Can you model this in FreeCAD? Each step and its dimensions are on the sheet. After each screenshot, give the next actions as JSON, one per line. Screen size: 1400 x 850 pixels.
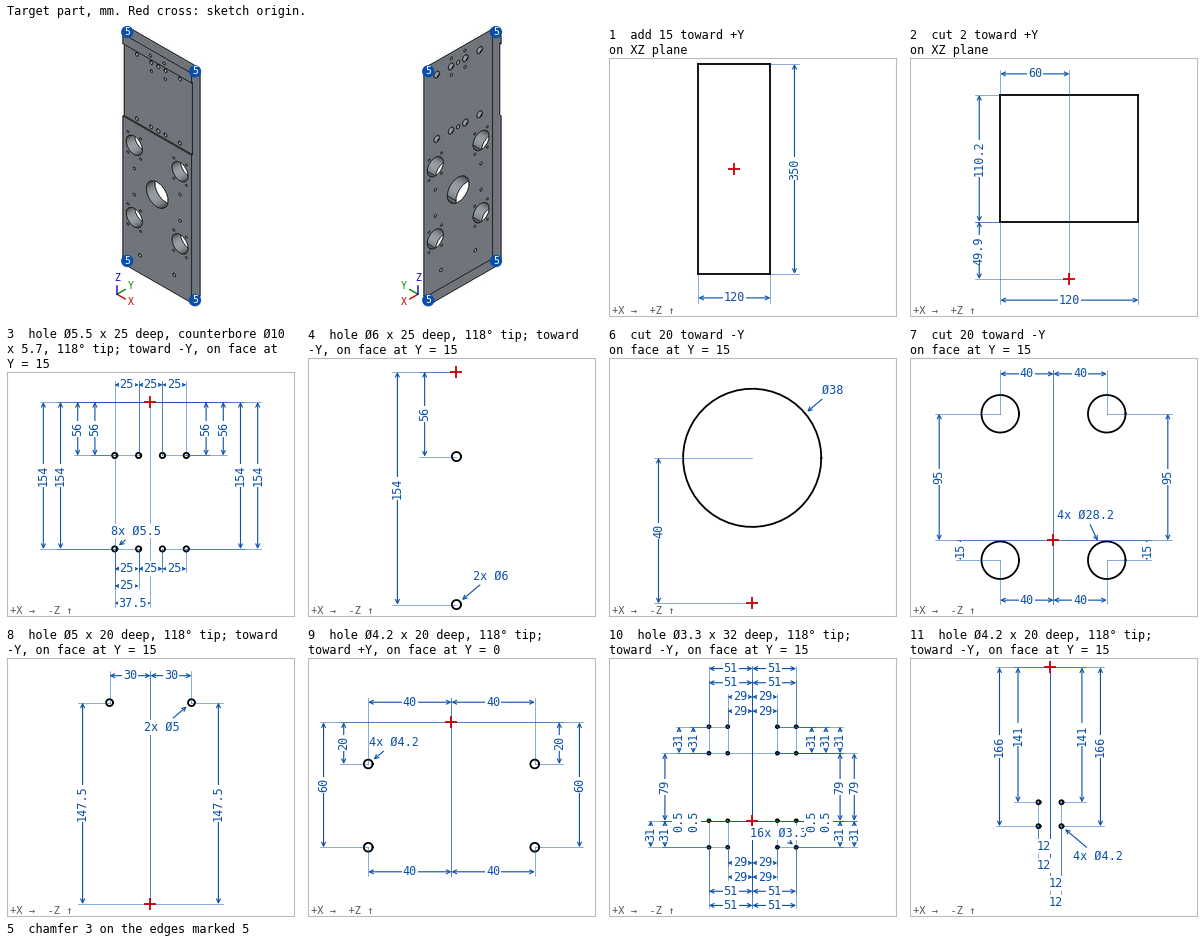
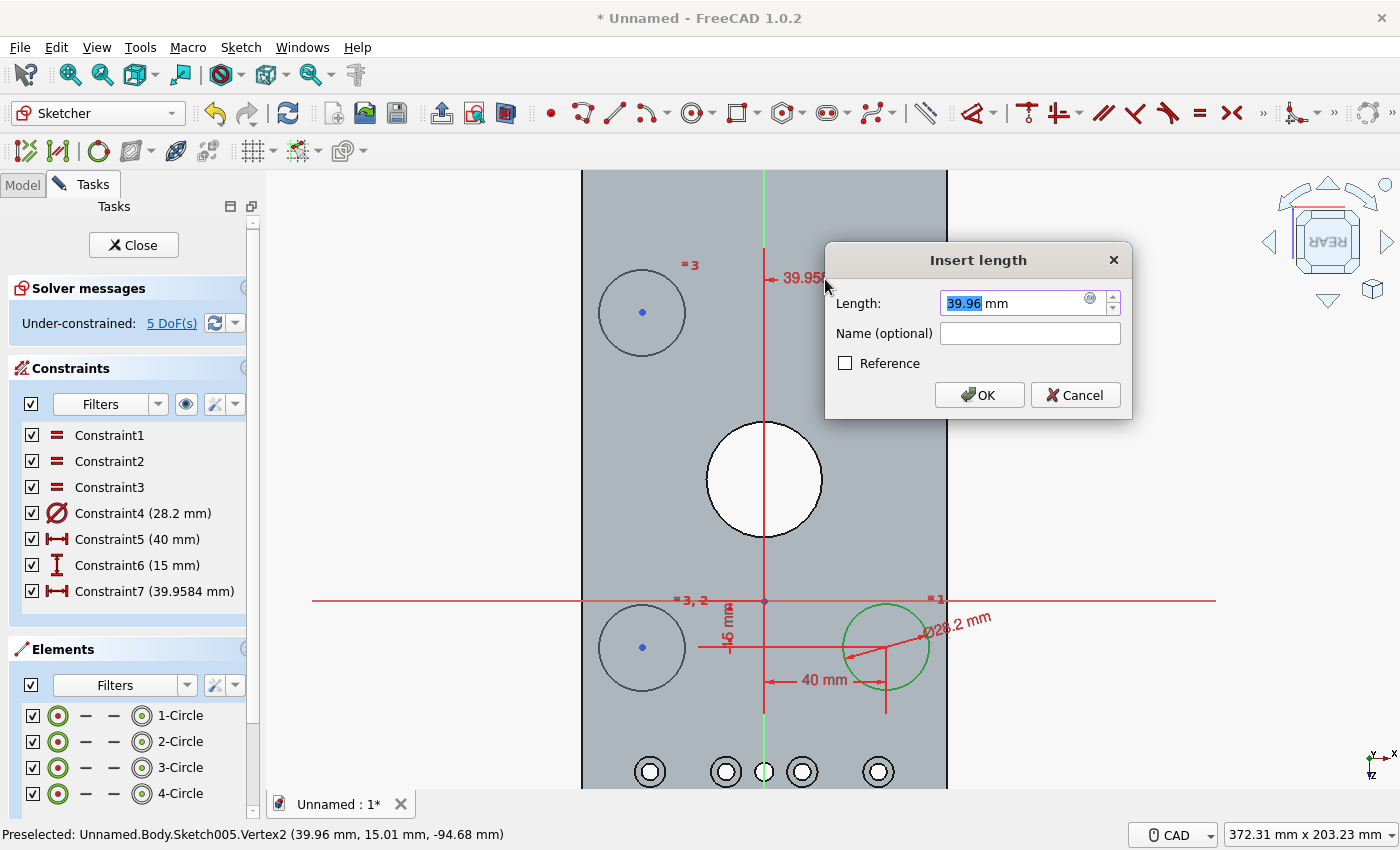
{"action": "type", "text": "40"}
{"action": "key", "text": "Return"}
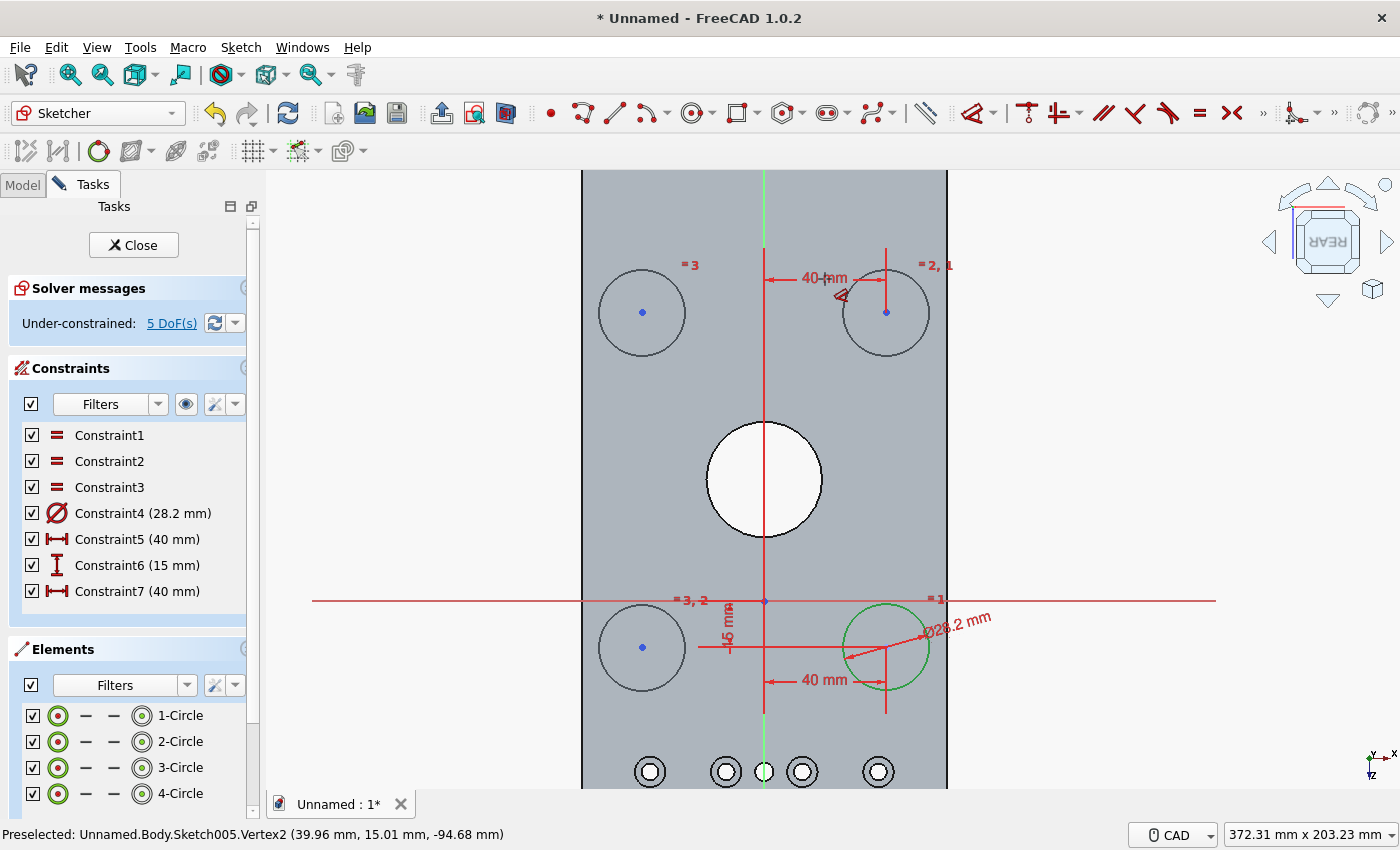
{"action": "left_click", "coordinate": [886, 313]}
{"action": "left_click", "coordinate": [920, 457]}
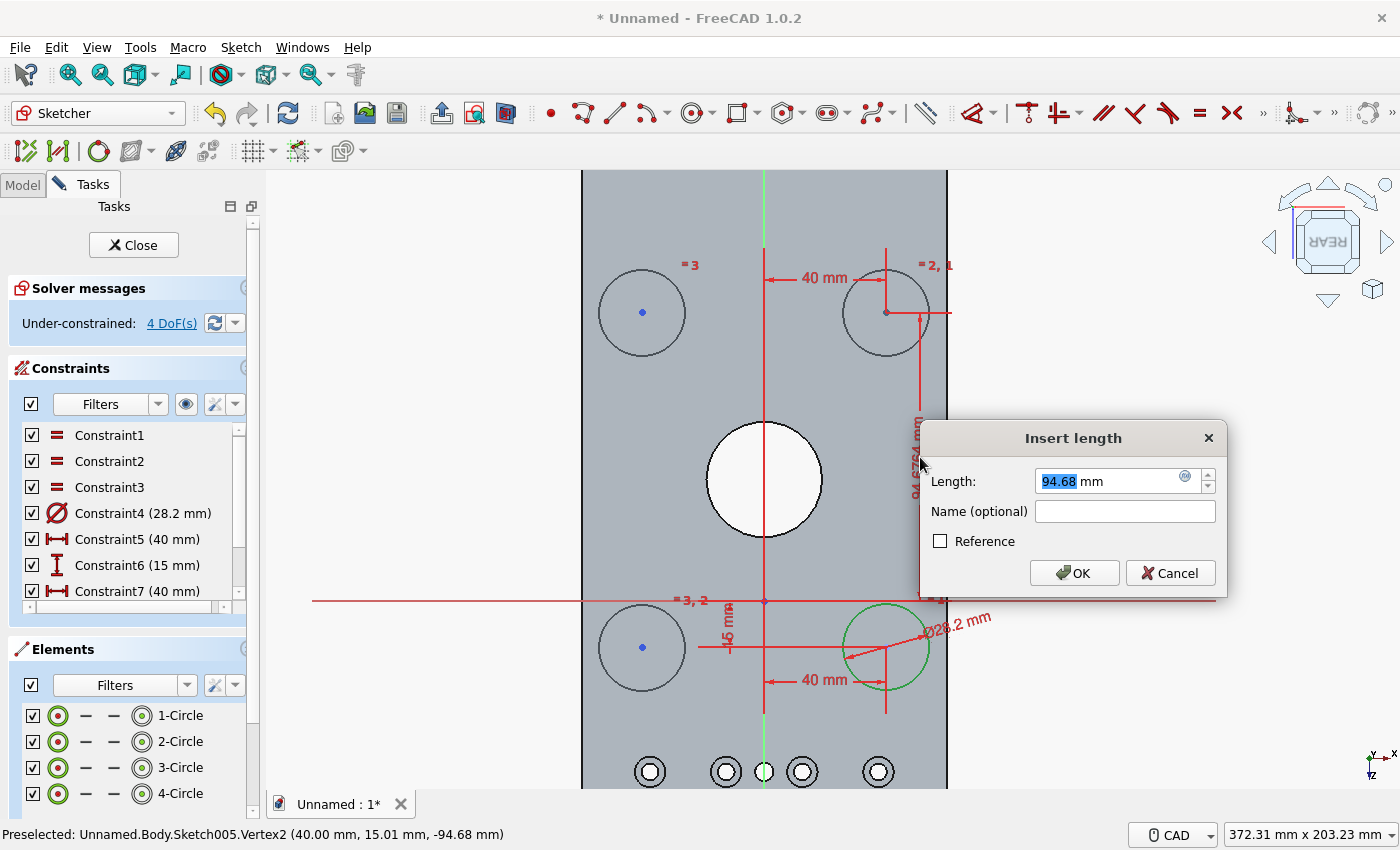
{"action": "type", "text": "95"}
{"action": "key", "text": "Return"}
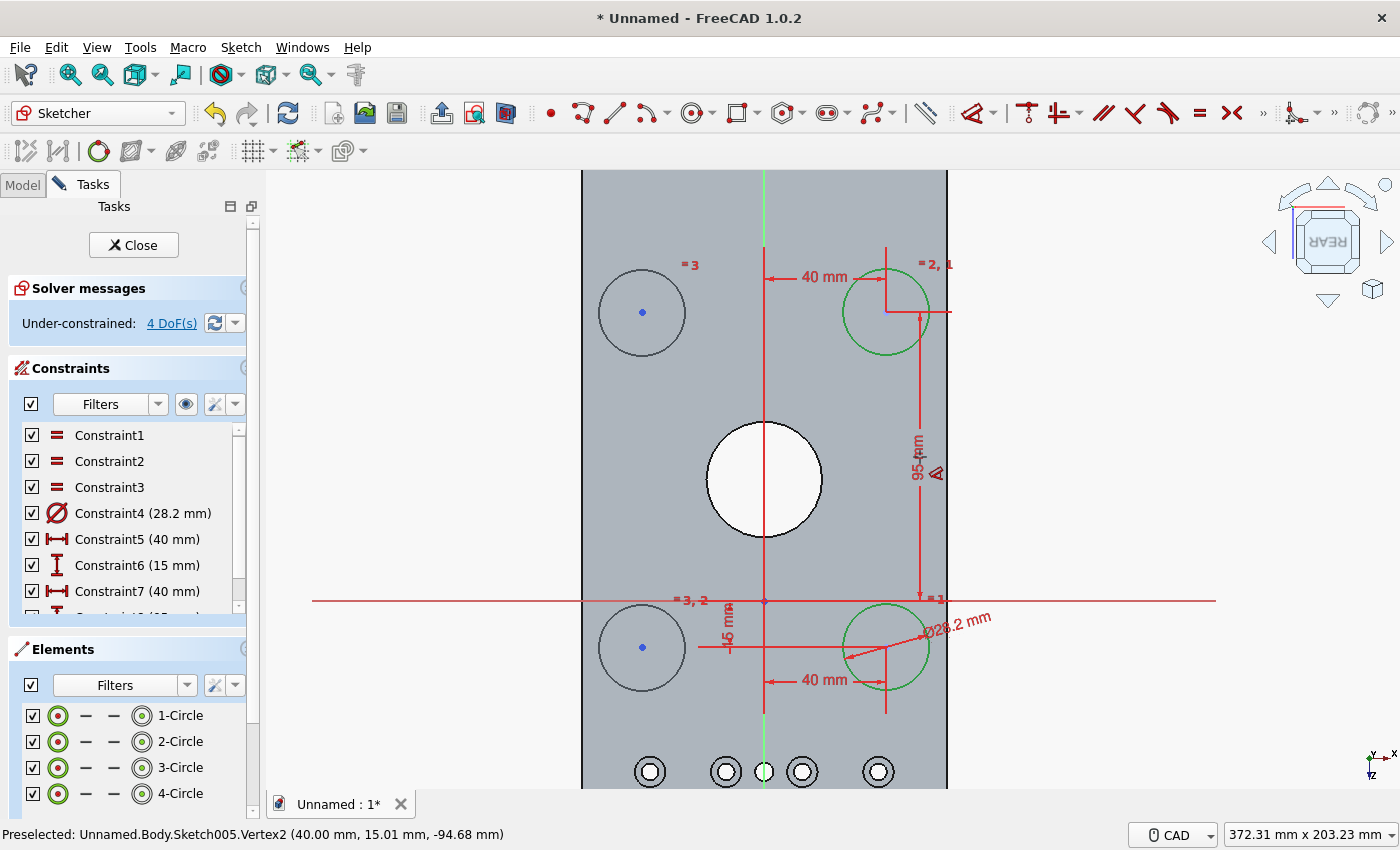
{"action": "left_click", "coordinate": [642, 648]}
{"action": "left_click", "coordinate": [703, 682]}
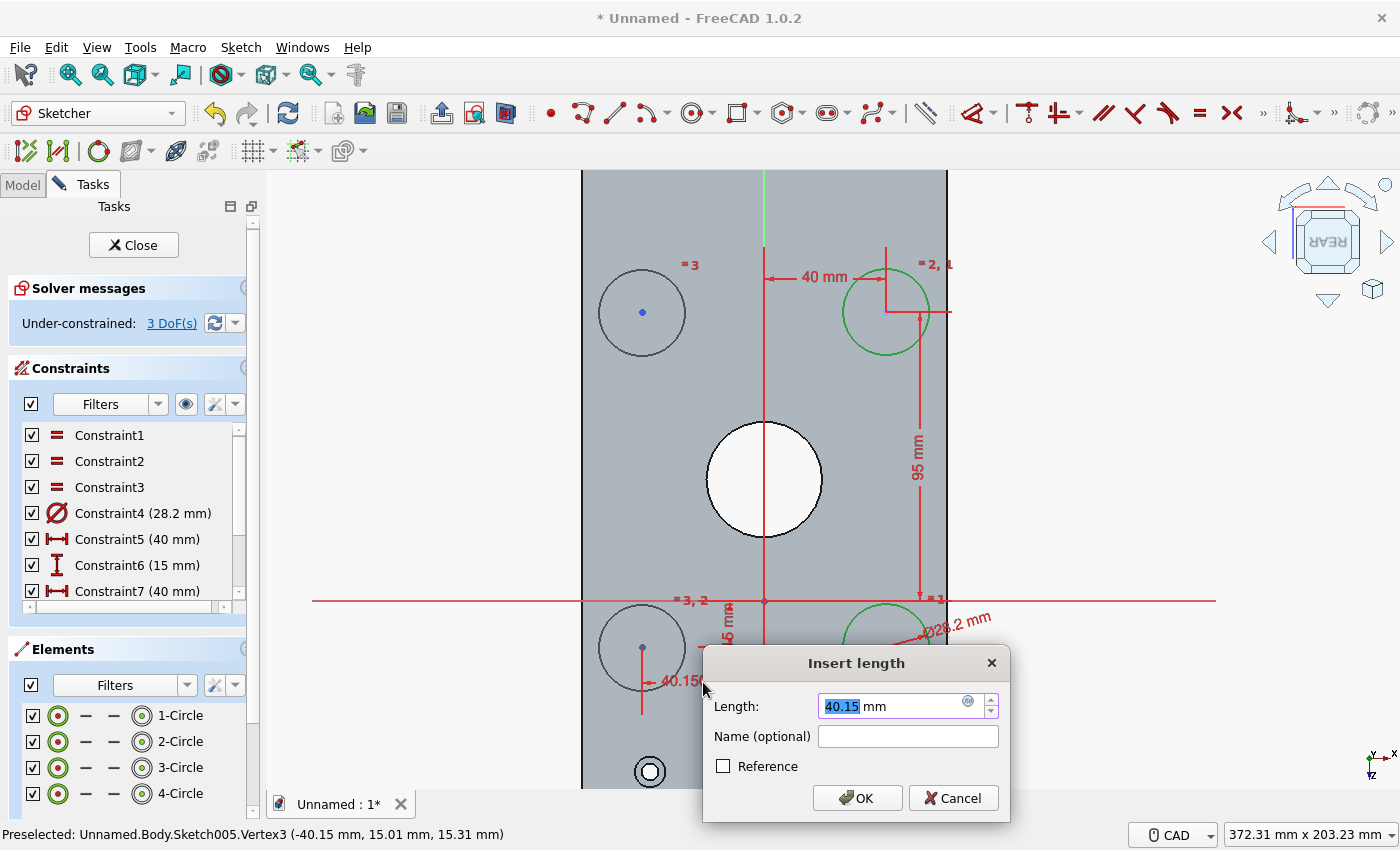
{"action": "type", "text": "40"}
{"action": "key", "text": "Return"}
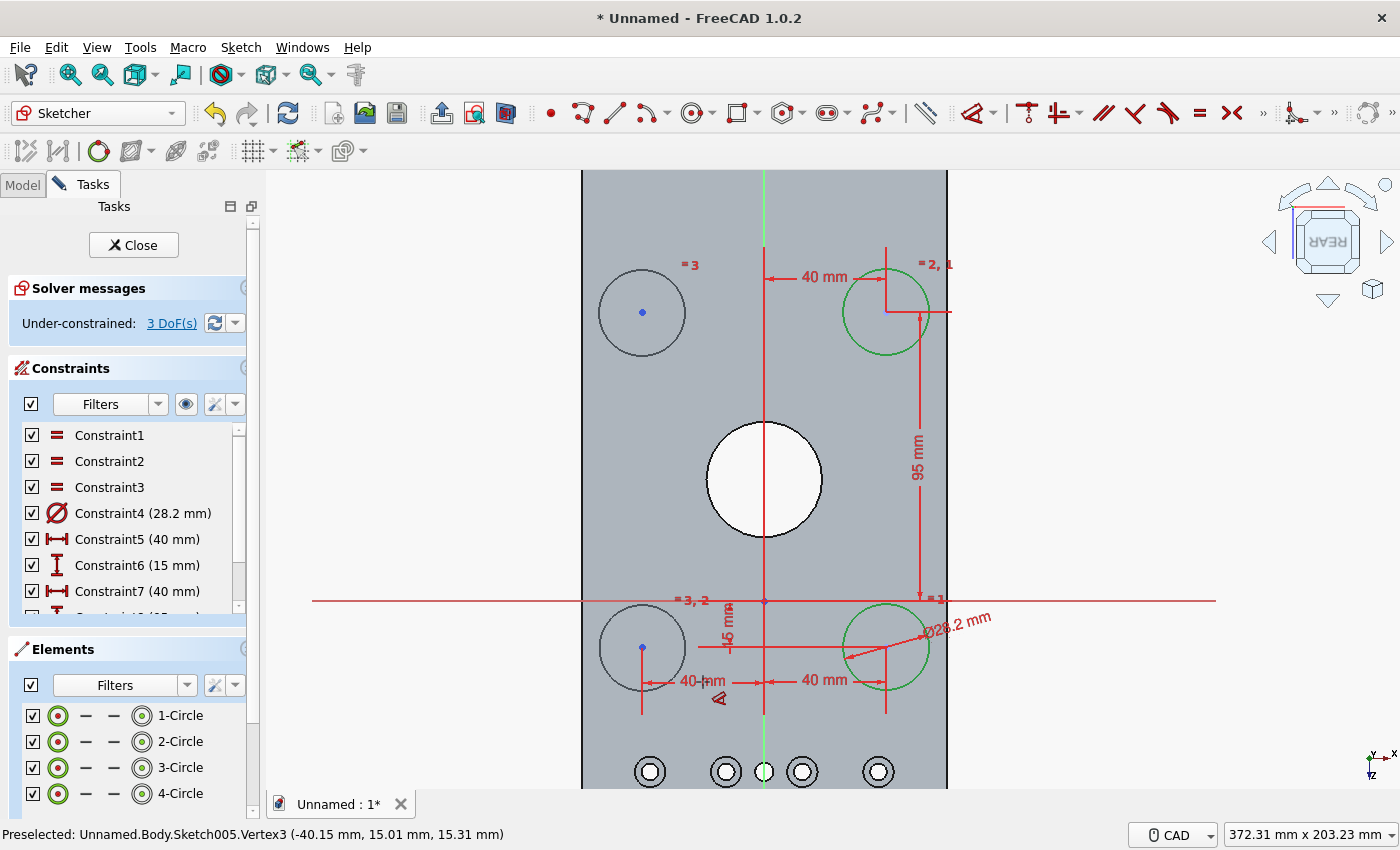
{"action": "left_click", "coordinate": [642, 648]}
{"action": "left_click", "coordinate": [584, 625]}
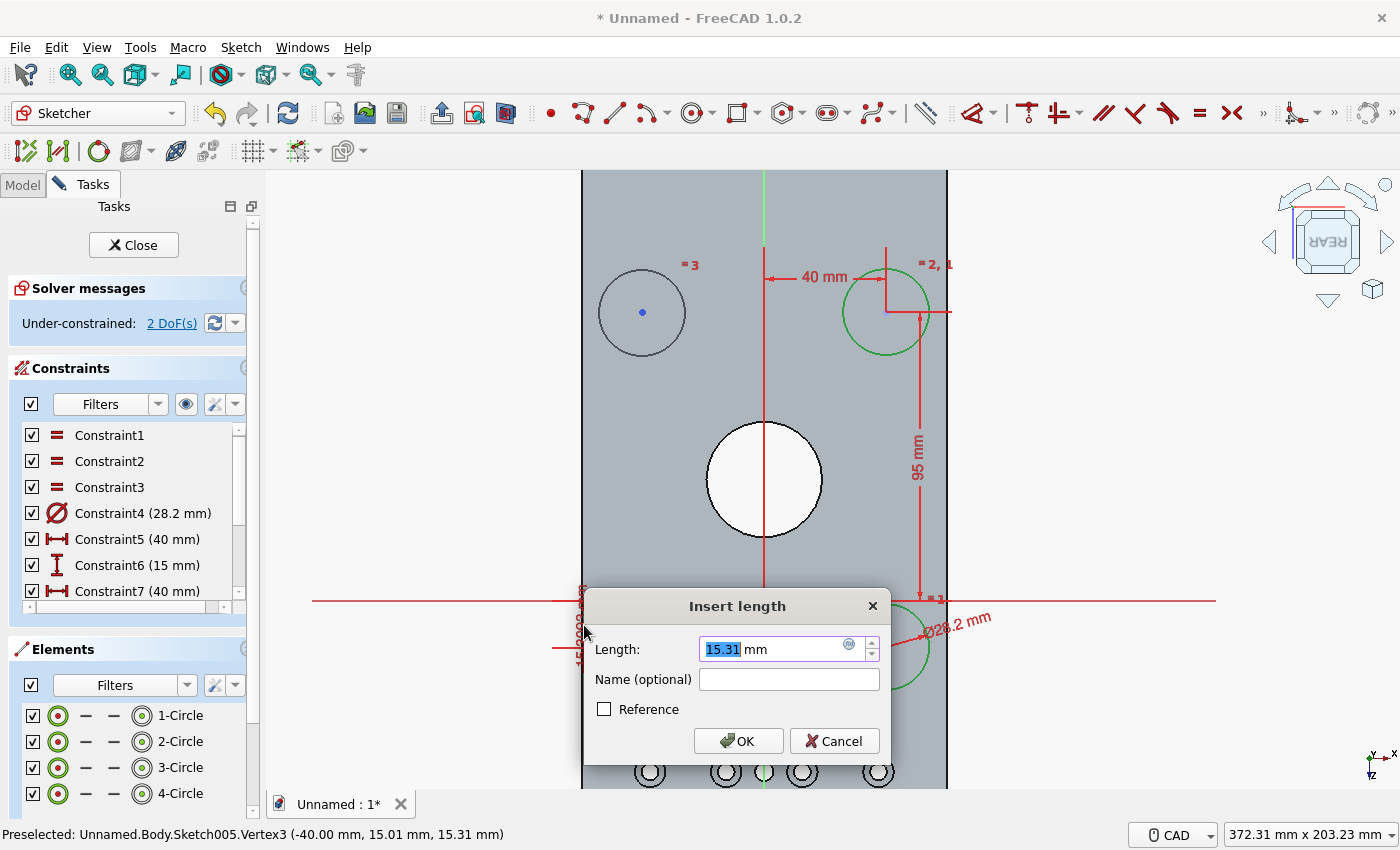
{"action": "type", "text": "15"}
{"action": "key", "text": "Return"}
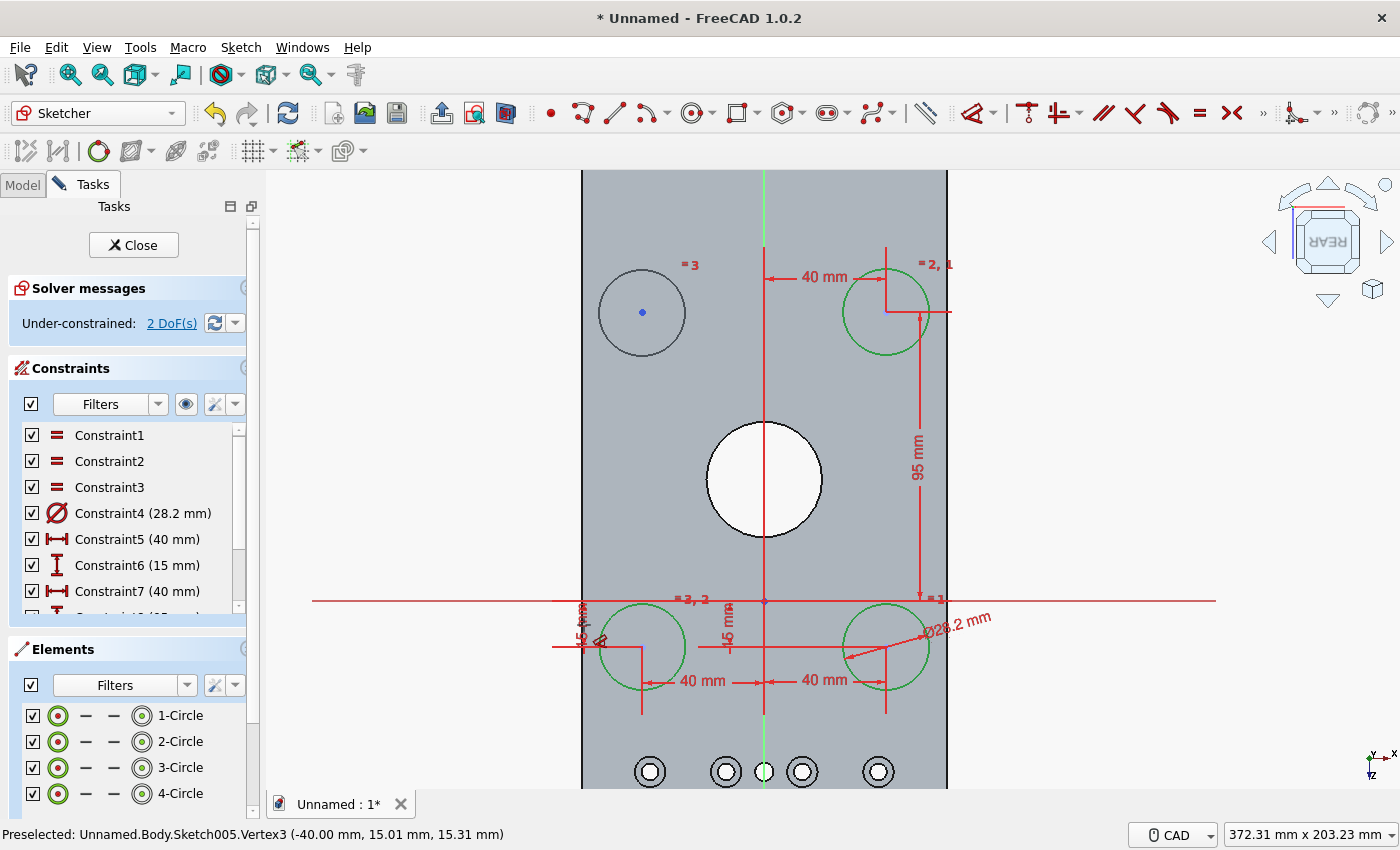
{"action": "left_click", "coordinate": [642, 313]}
{"action": "left_click", "coordinate": [703, 279]}